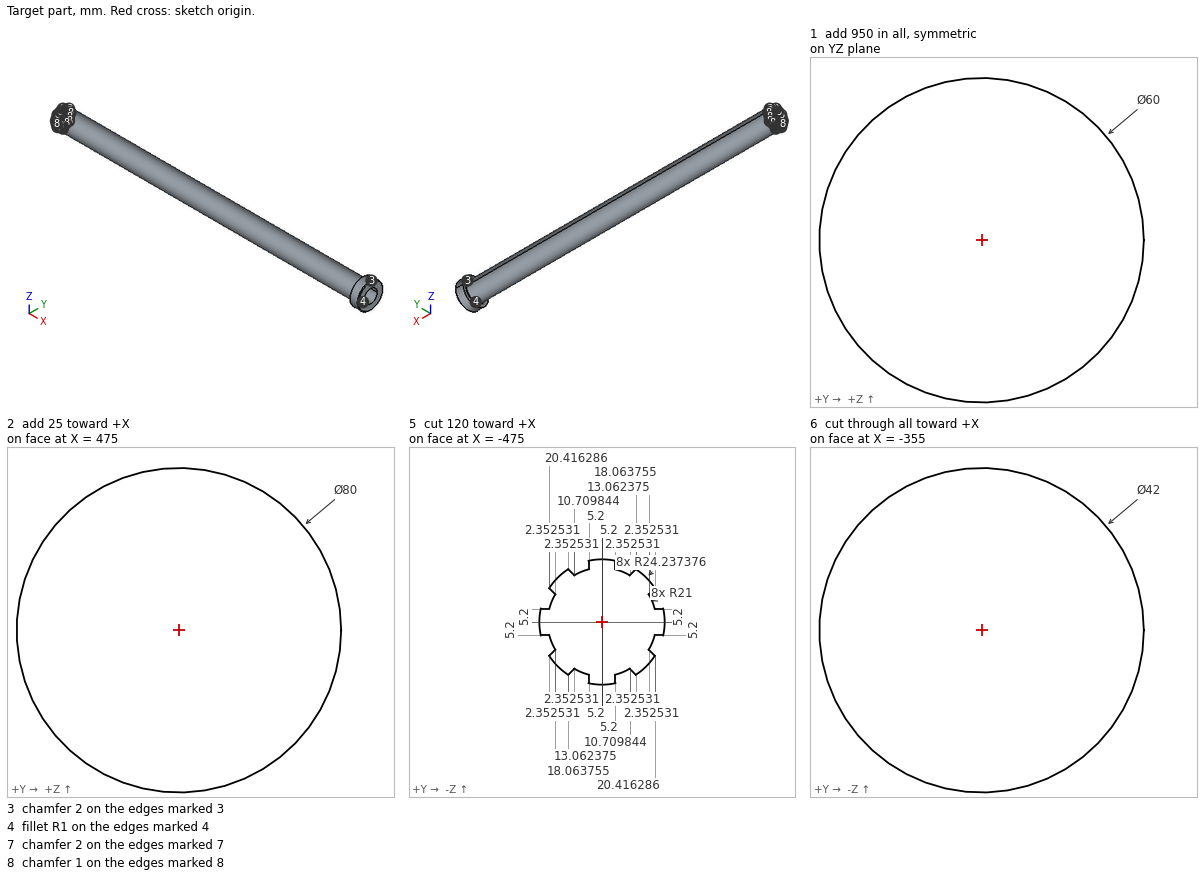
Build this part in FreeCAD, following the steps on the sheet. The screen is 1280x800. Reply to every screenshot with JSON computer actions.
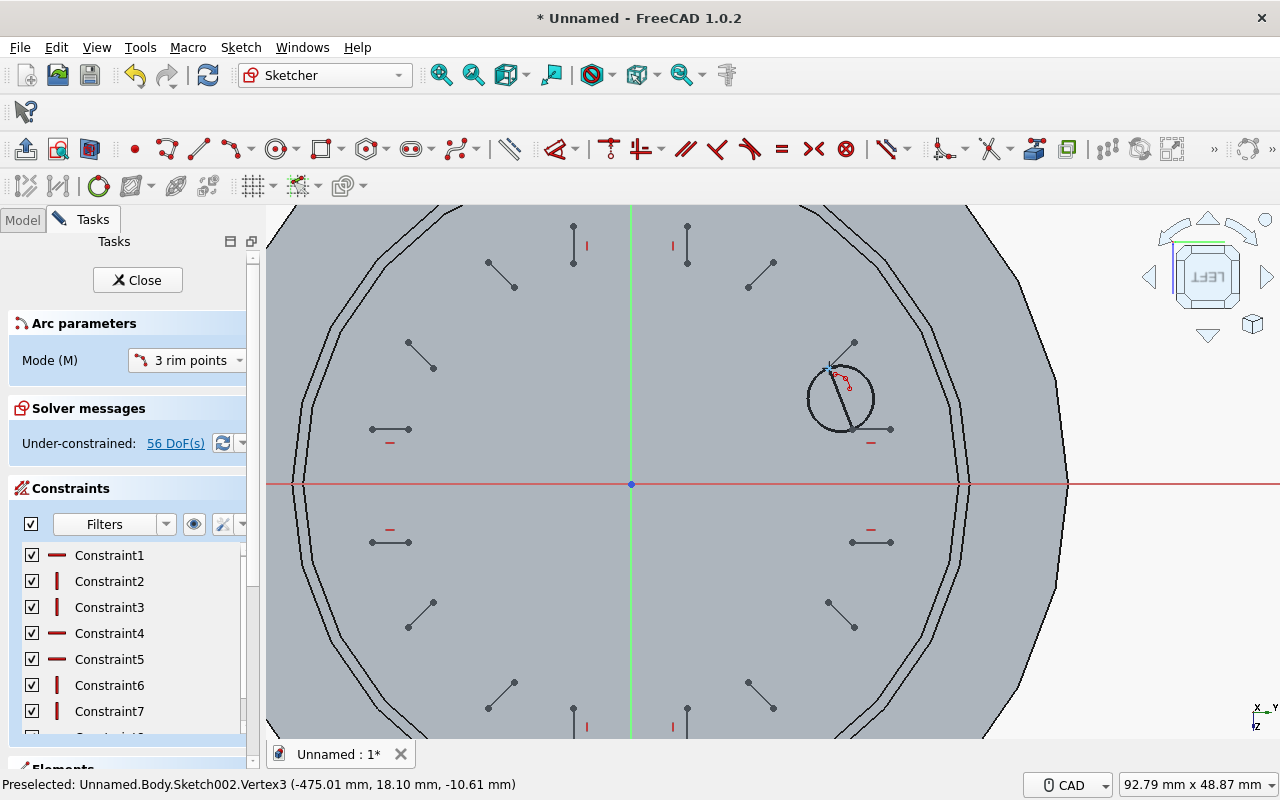
{"action": "scroll", "coordinate": [843, 396], "scroll_direction": "up", "scroll_amount": 10}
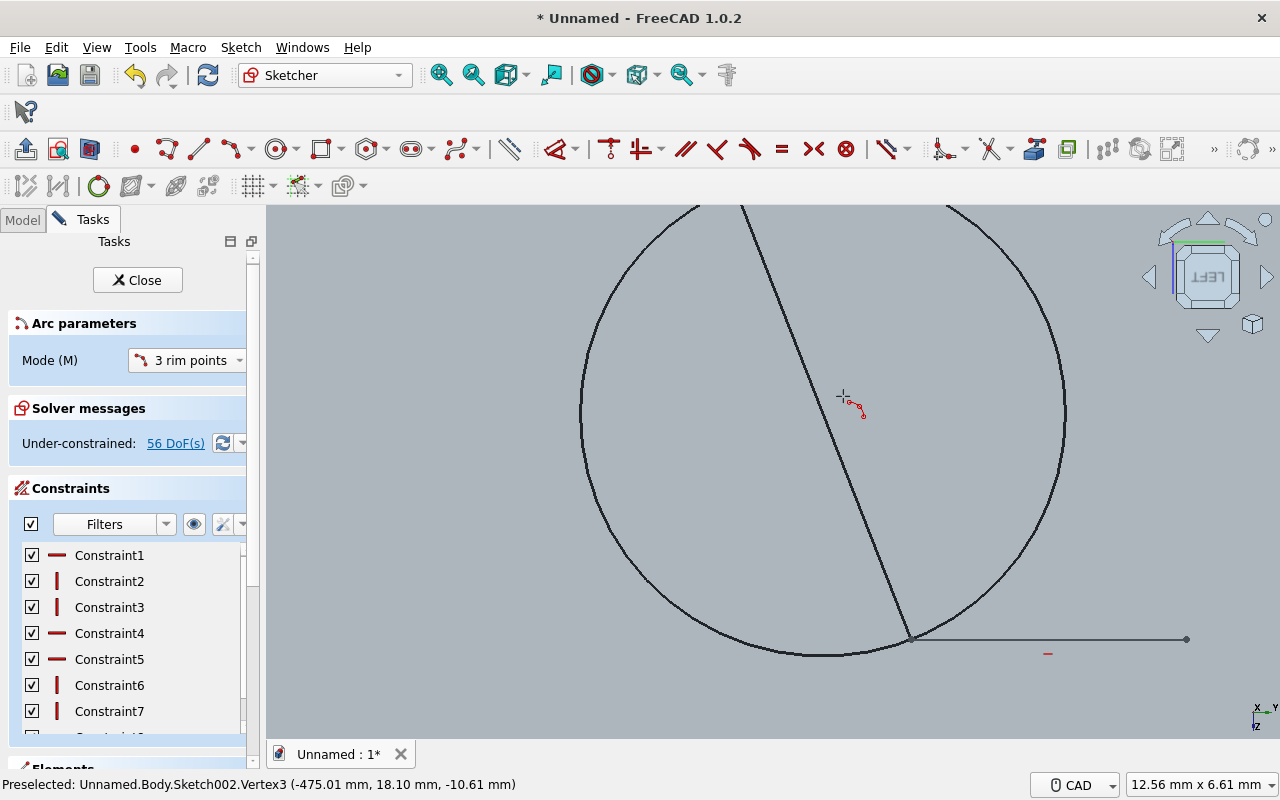
{"action": "left_click", "coordinate": [840, 396]}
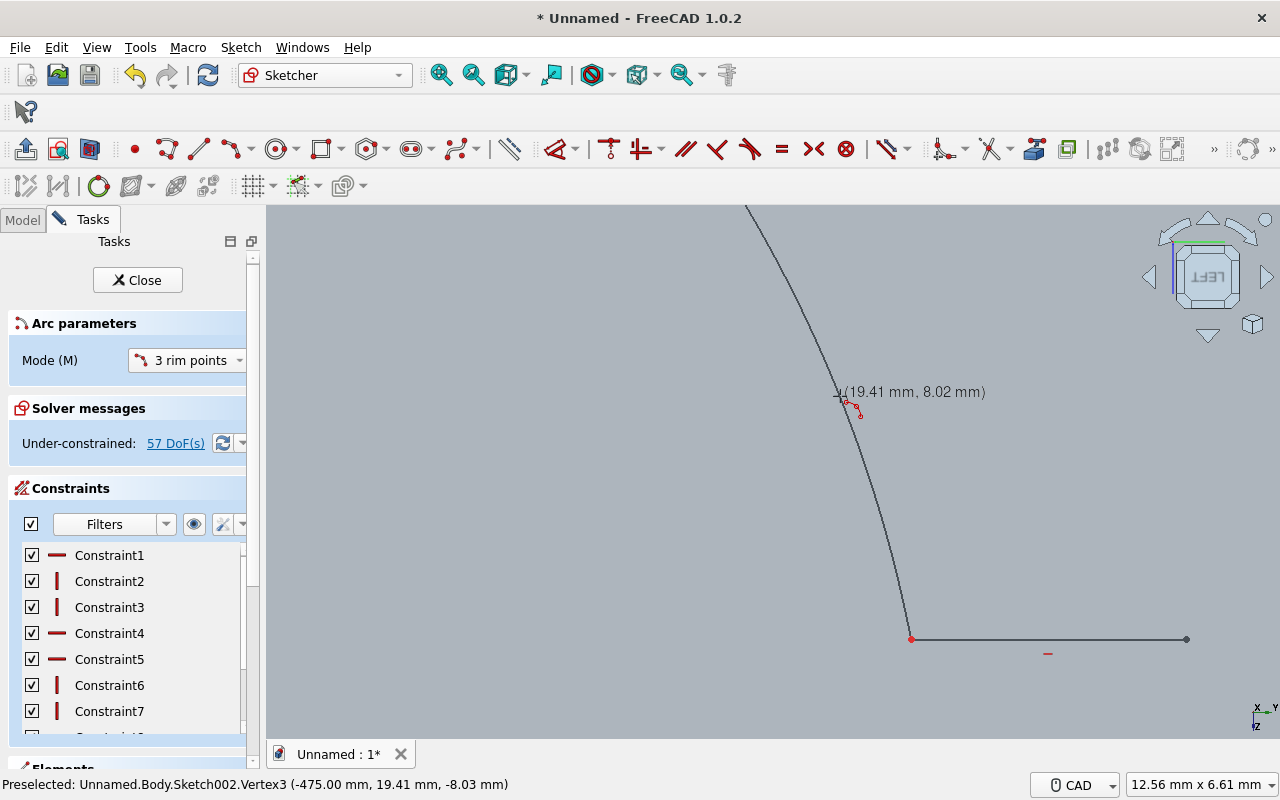
{"action": "scroll", "coordinate": [847, 415], "scroll_direction": "down", "scroll_amount": 12}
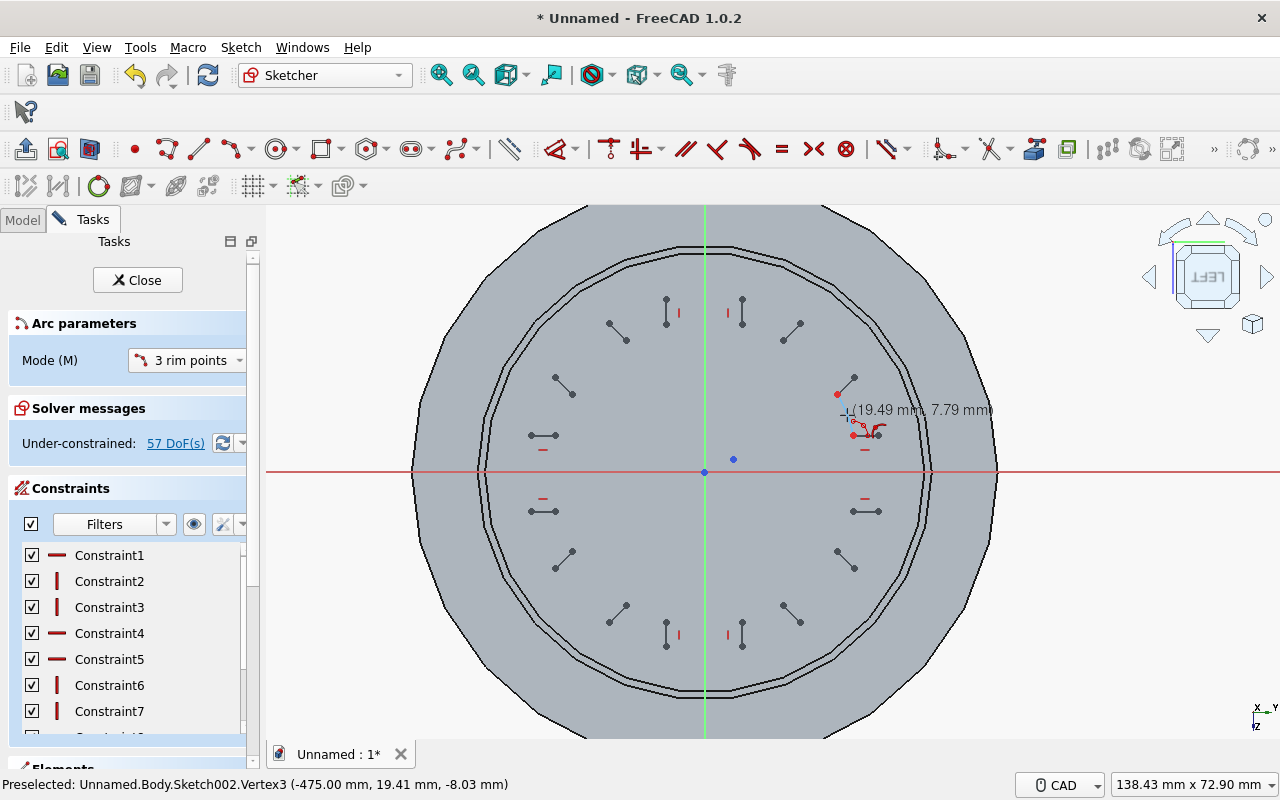
{"action": "scroll", "coordinate": [854, 377], "scroll_direction": "up", "scroll_amount": 2}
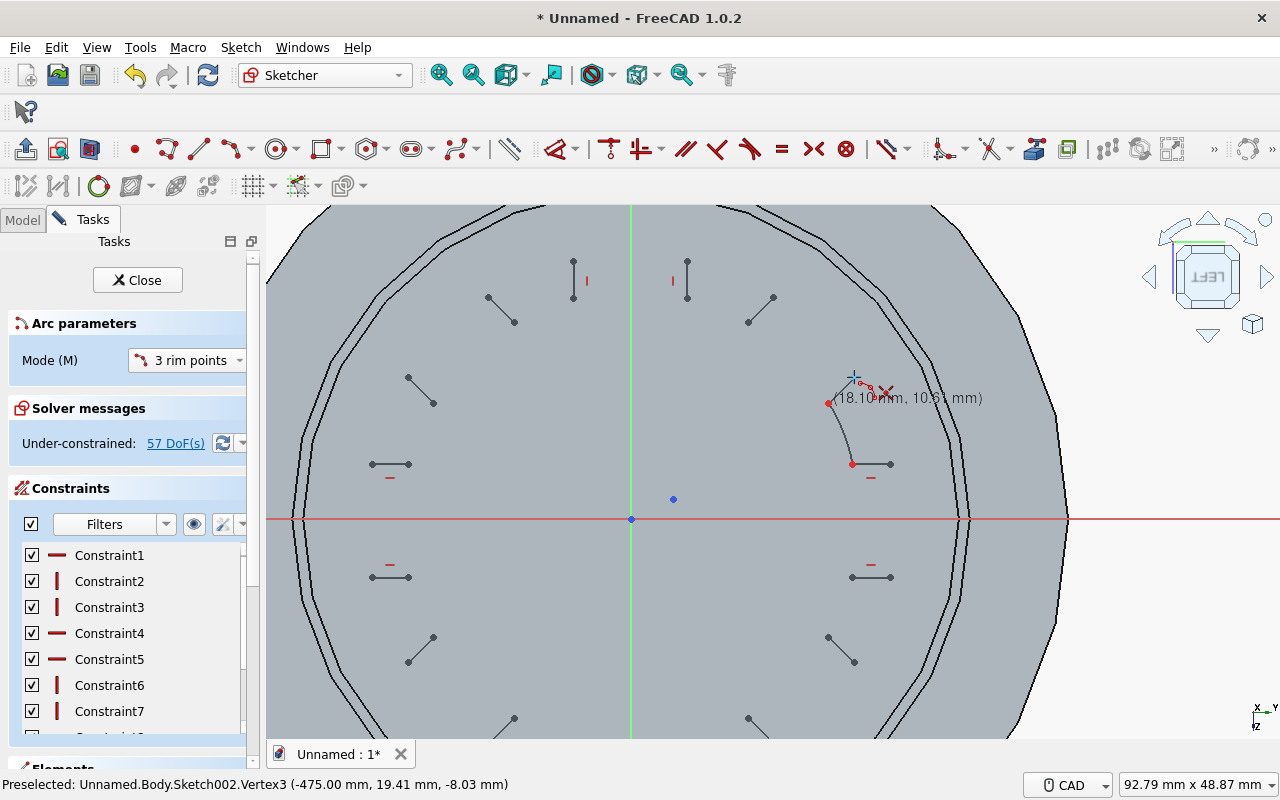
{"action": "left_click", "coordinate": [854, 378]}
{"action": "left_click", "coordinate": [774, 297]}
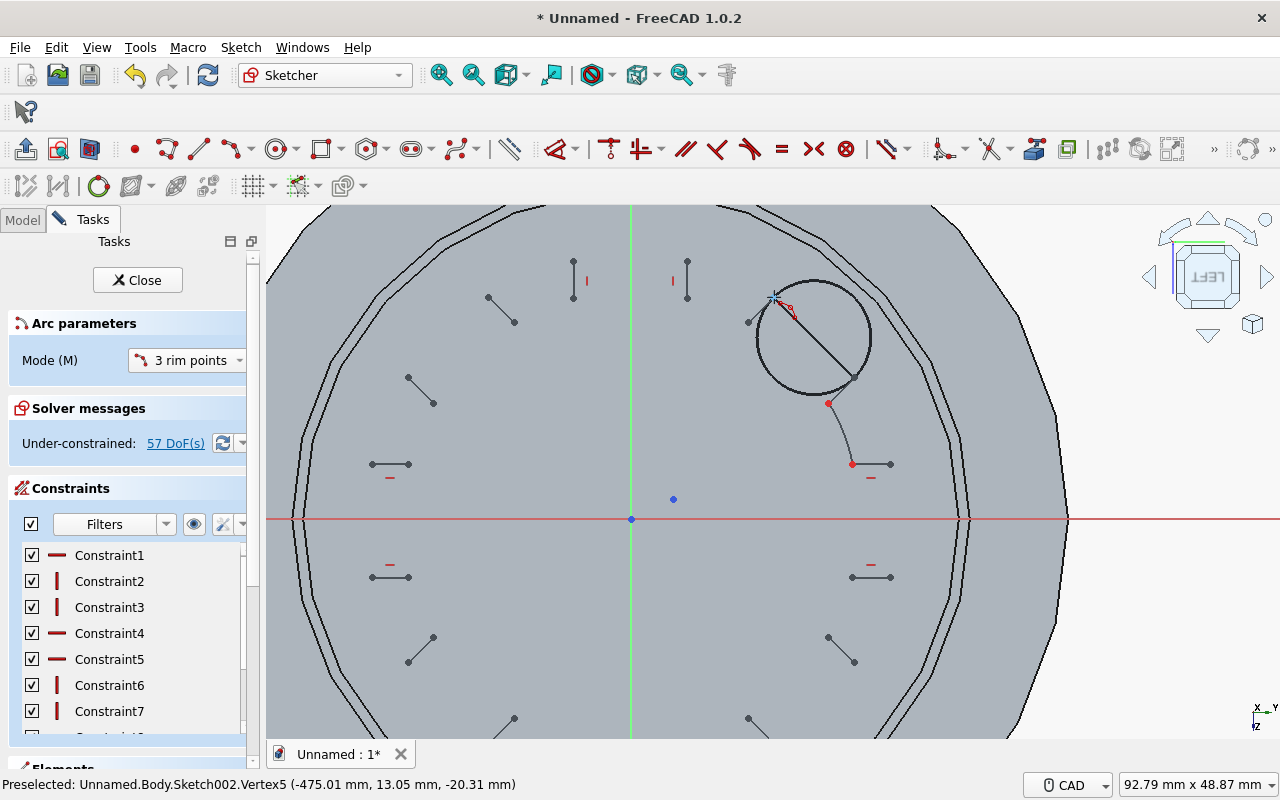
{"action": "scroll", "coordinate": [818, 332], "scroll_direction": "up", "scroll_amount": 5}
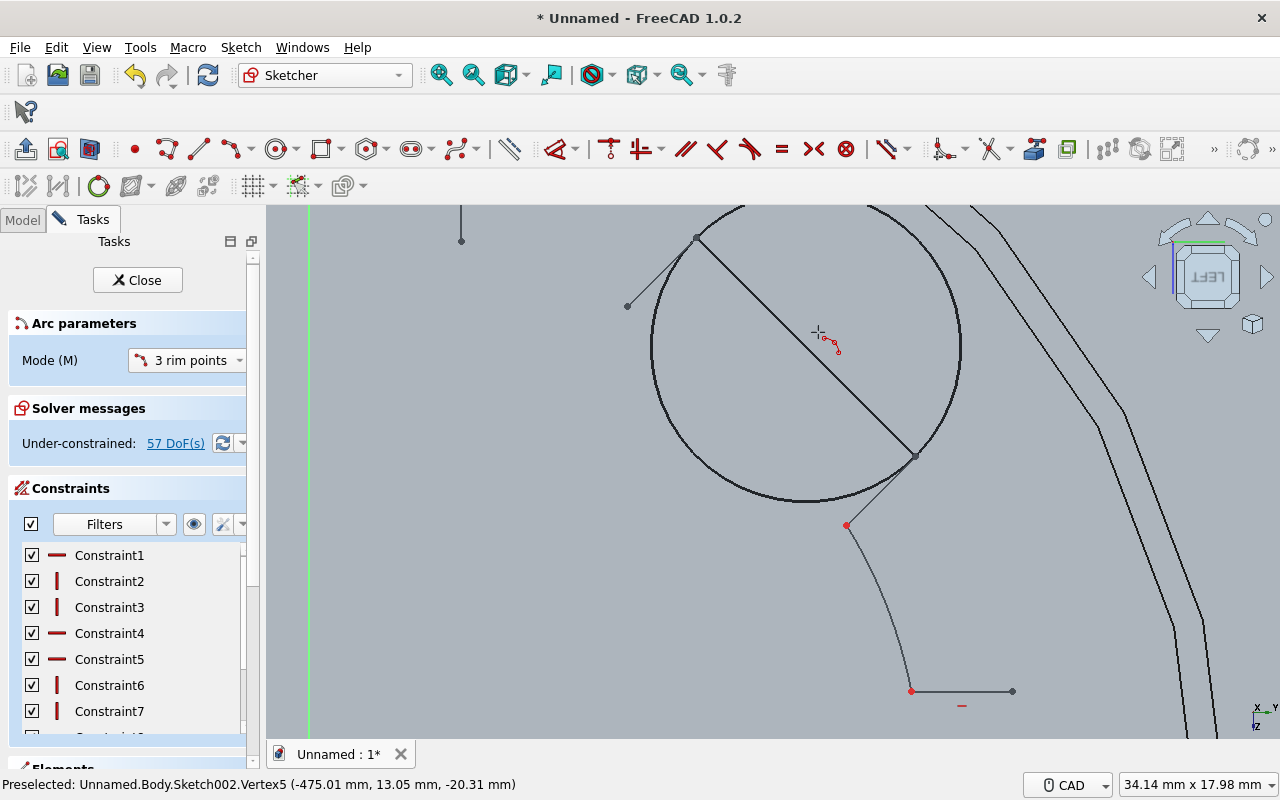
{"action": "left_click", "coordinate": [818, 332]}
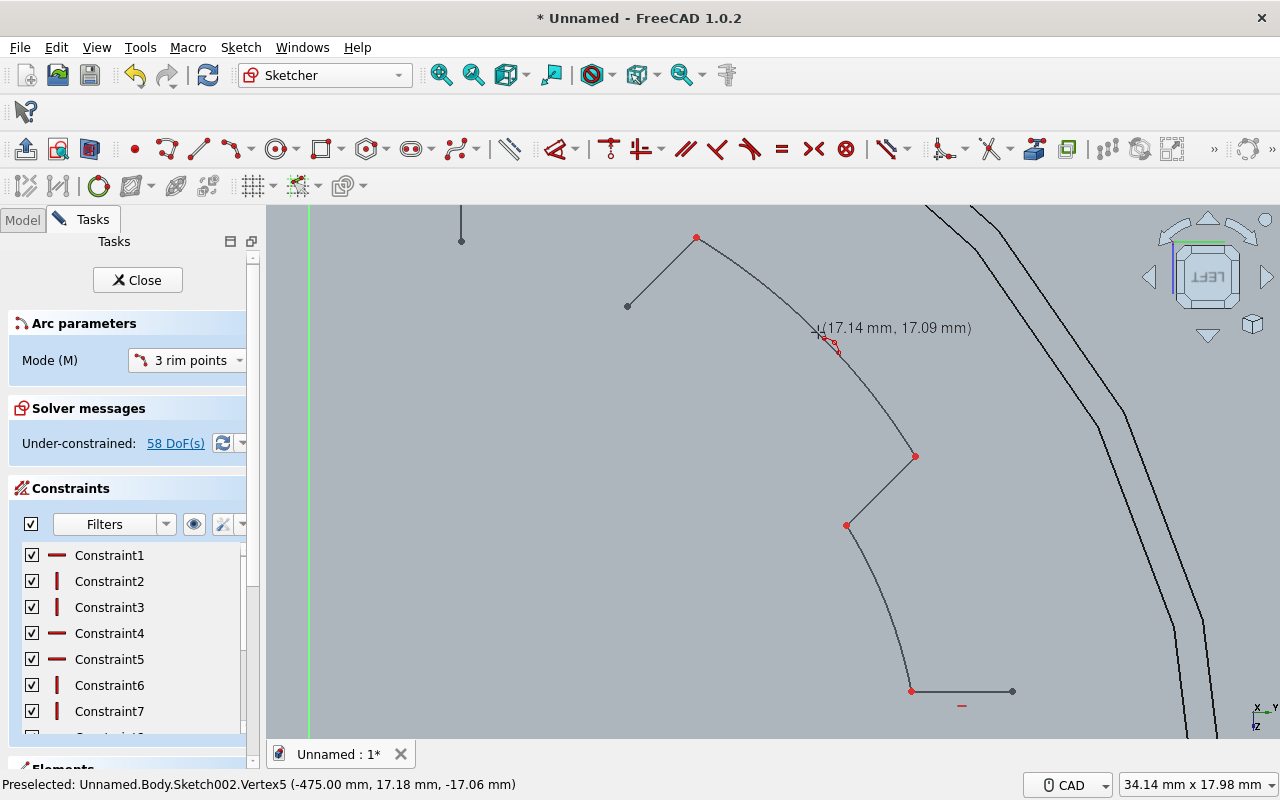
{"action": "scroll", "coordinate": [834, 351], "scroll_direction": "down", "scroll_amount": 7}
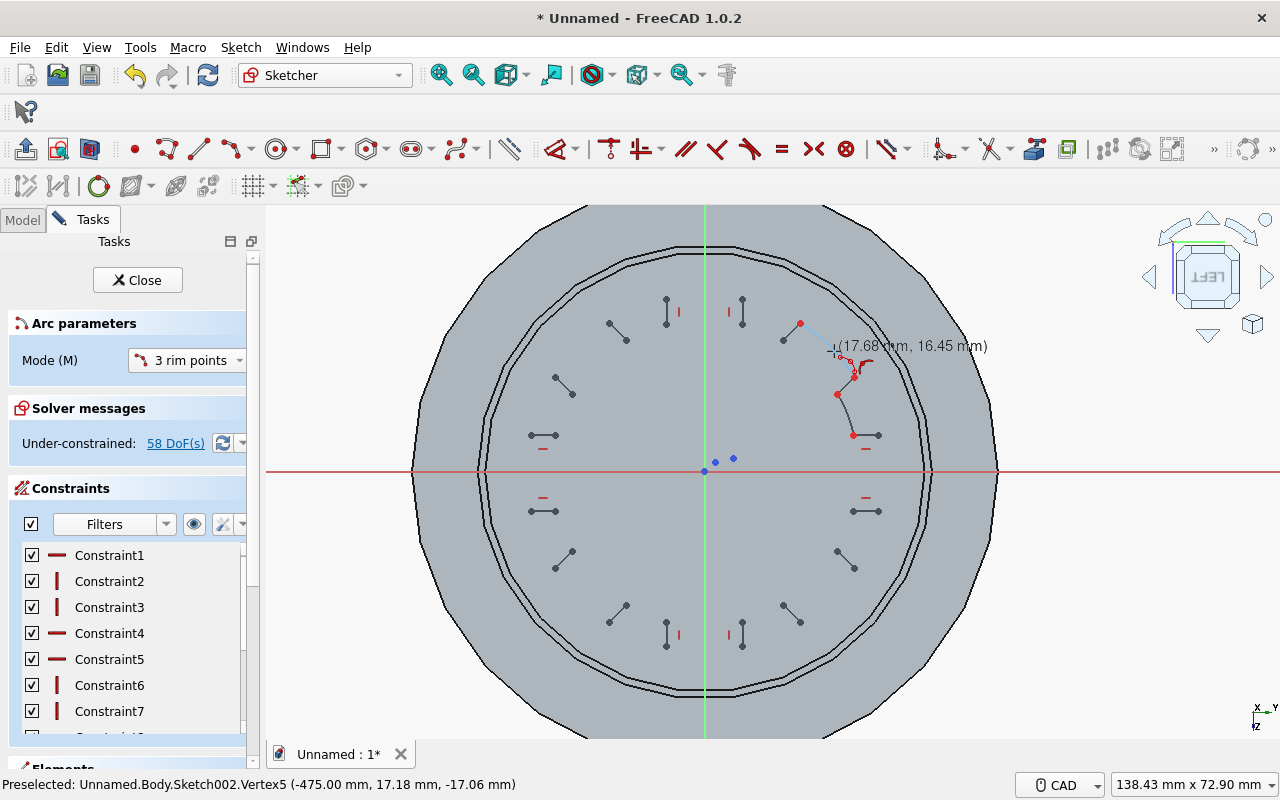
{"action": "scroll", "coordinate": [783, 340], "scroll_direction": "up", "scroll_amount": 2}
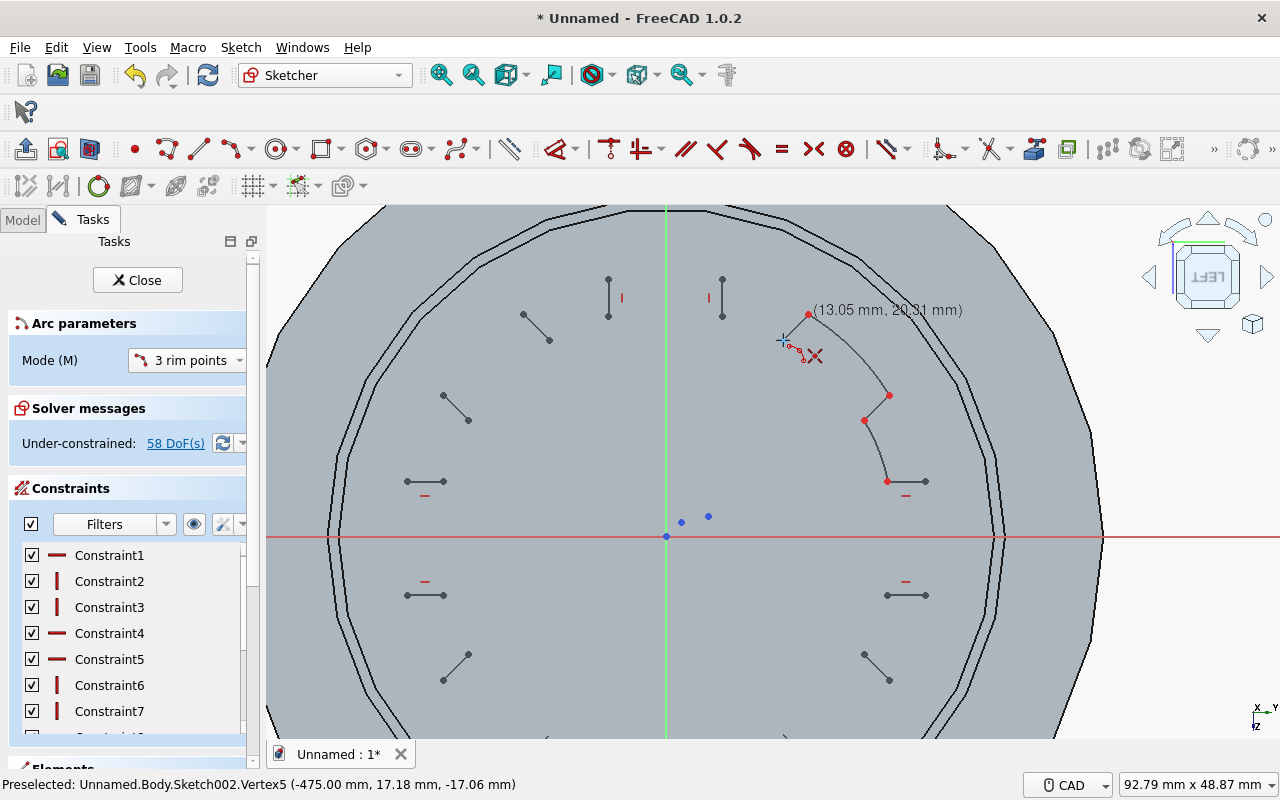
{"action": "left_click", "coordinate": [784, 340]}
{"action": "left_click", "coordinate": [722, 316]}